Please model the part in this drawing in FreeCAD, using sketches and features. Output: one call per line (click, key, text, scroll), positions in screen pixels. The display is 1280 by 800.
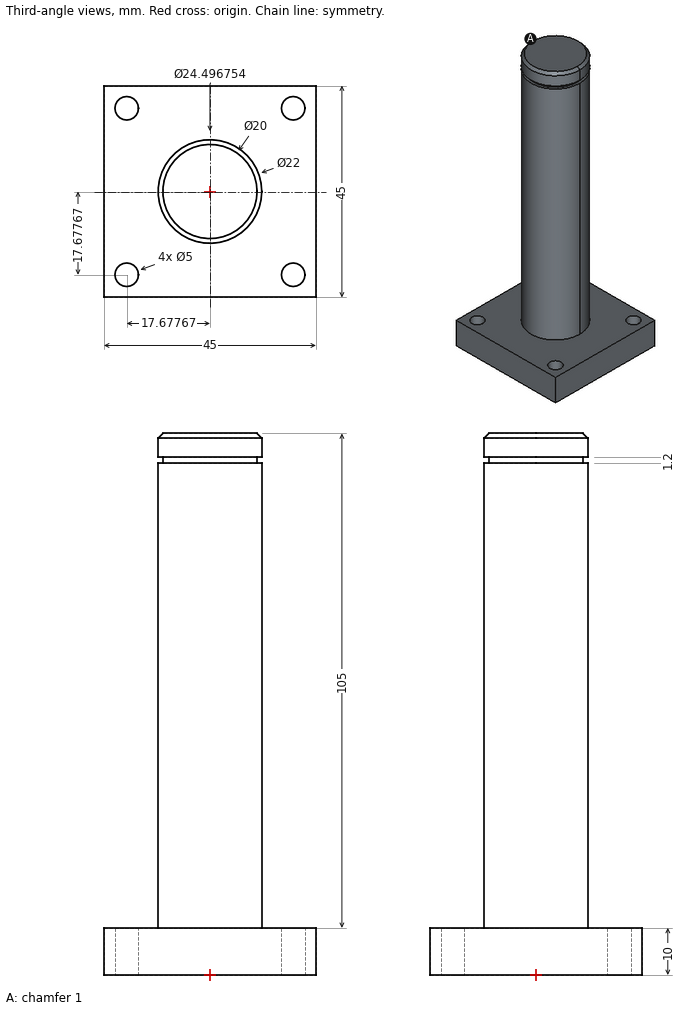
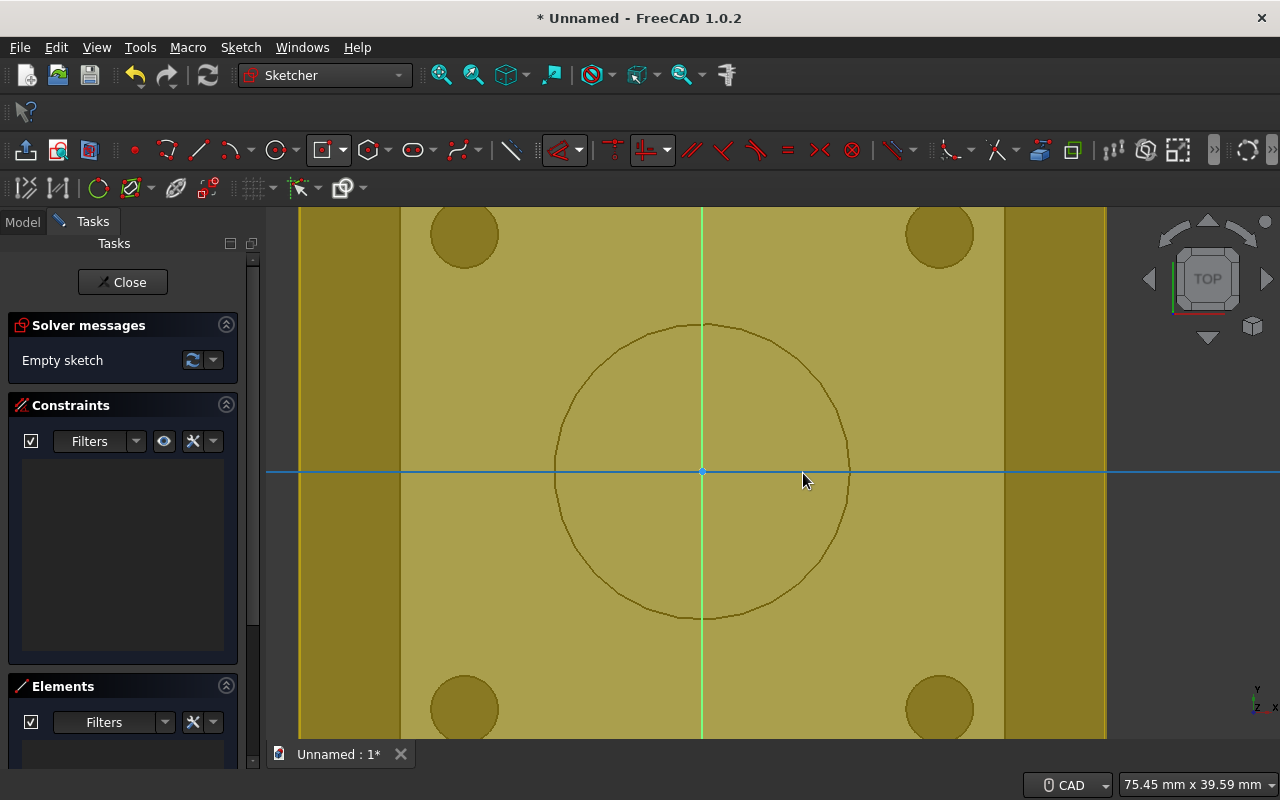
click(276, 150)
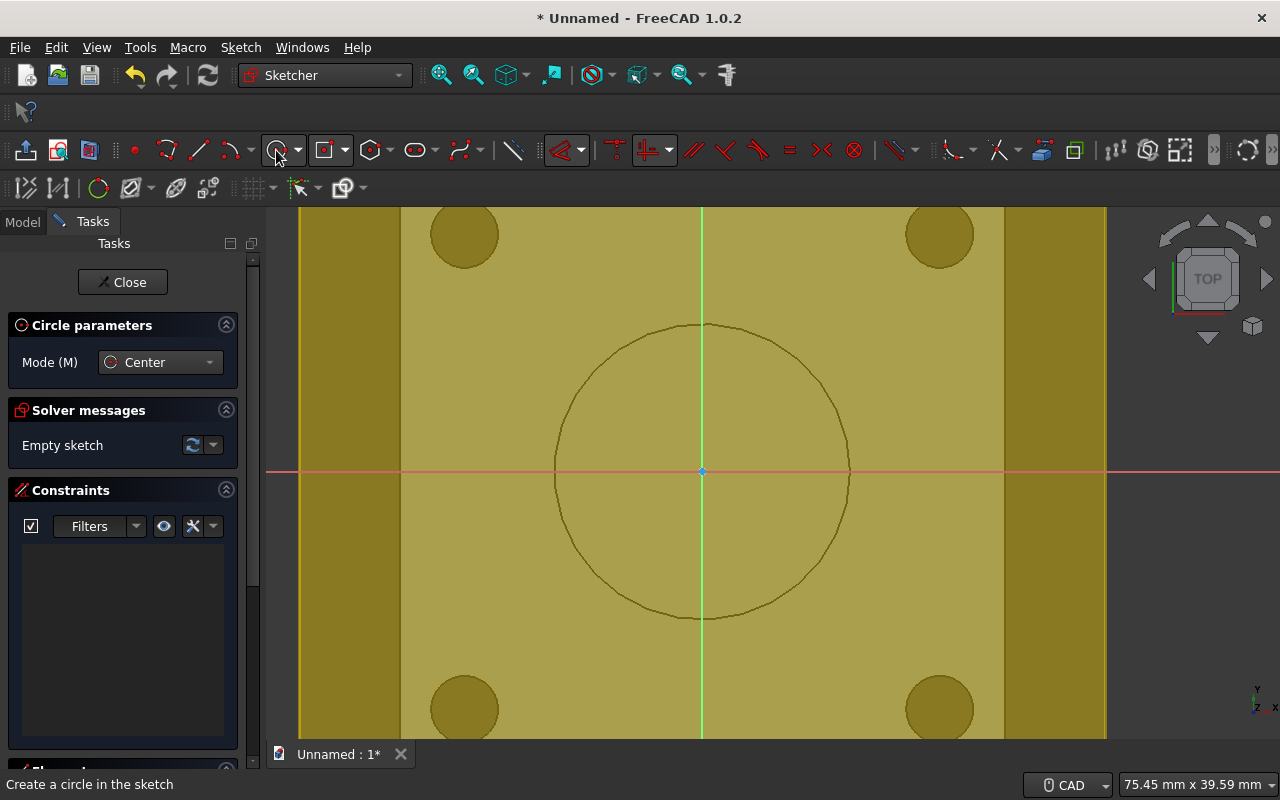
click(702, 472)
move(819, 355)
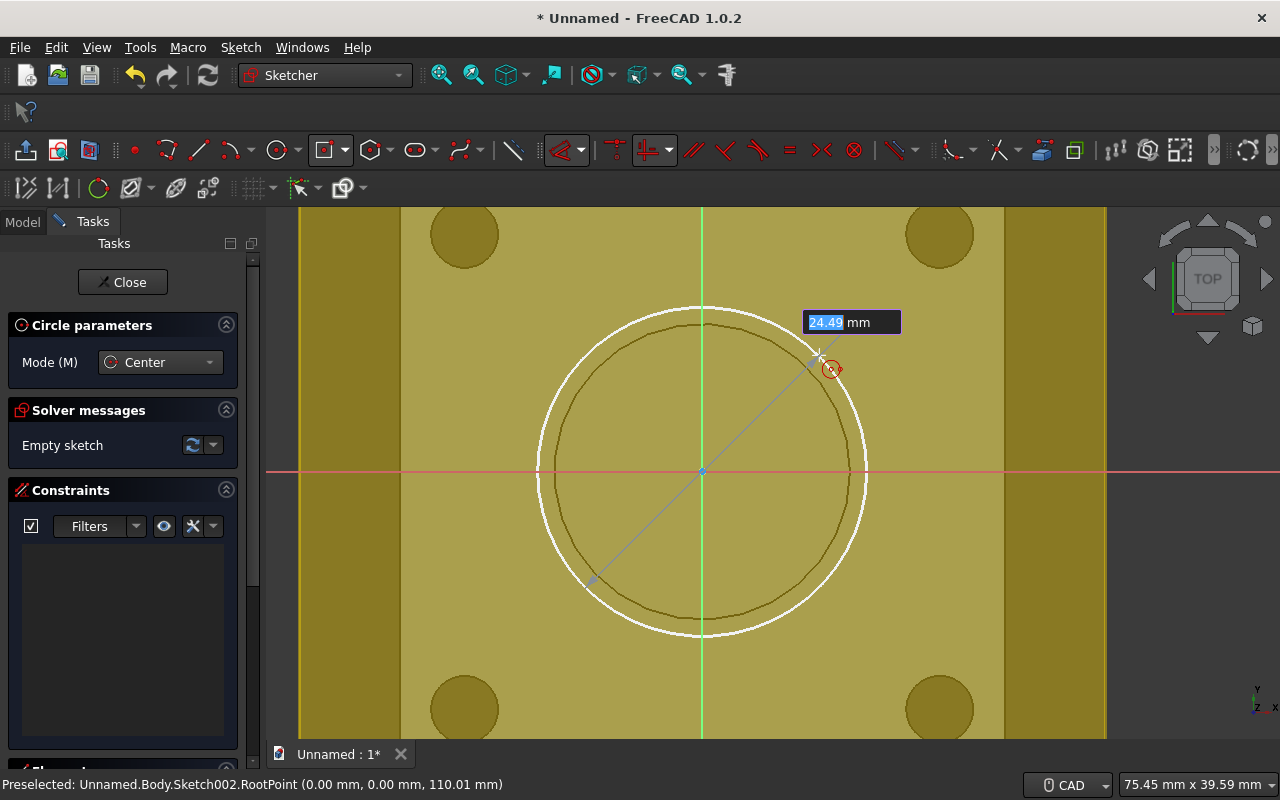
text(24.496754)
key(Return)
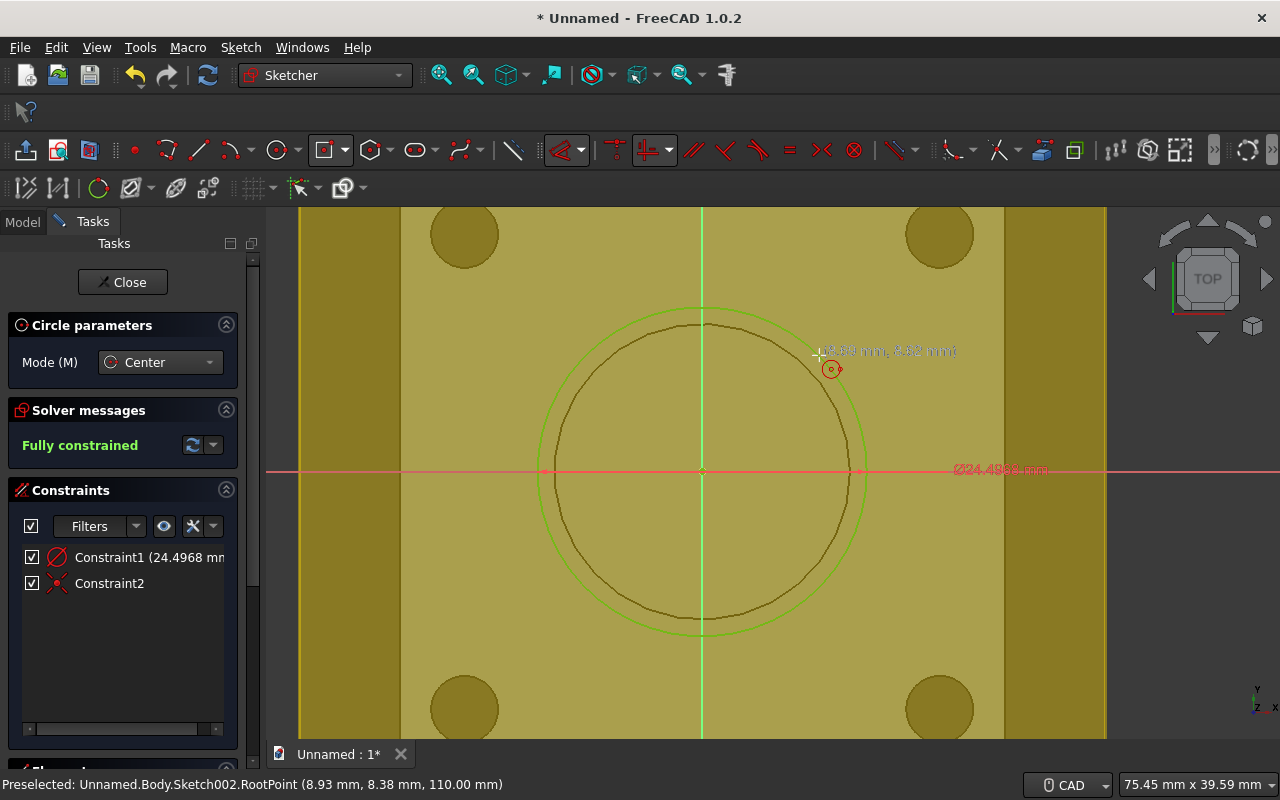
click(702, 472)
move(797, 377)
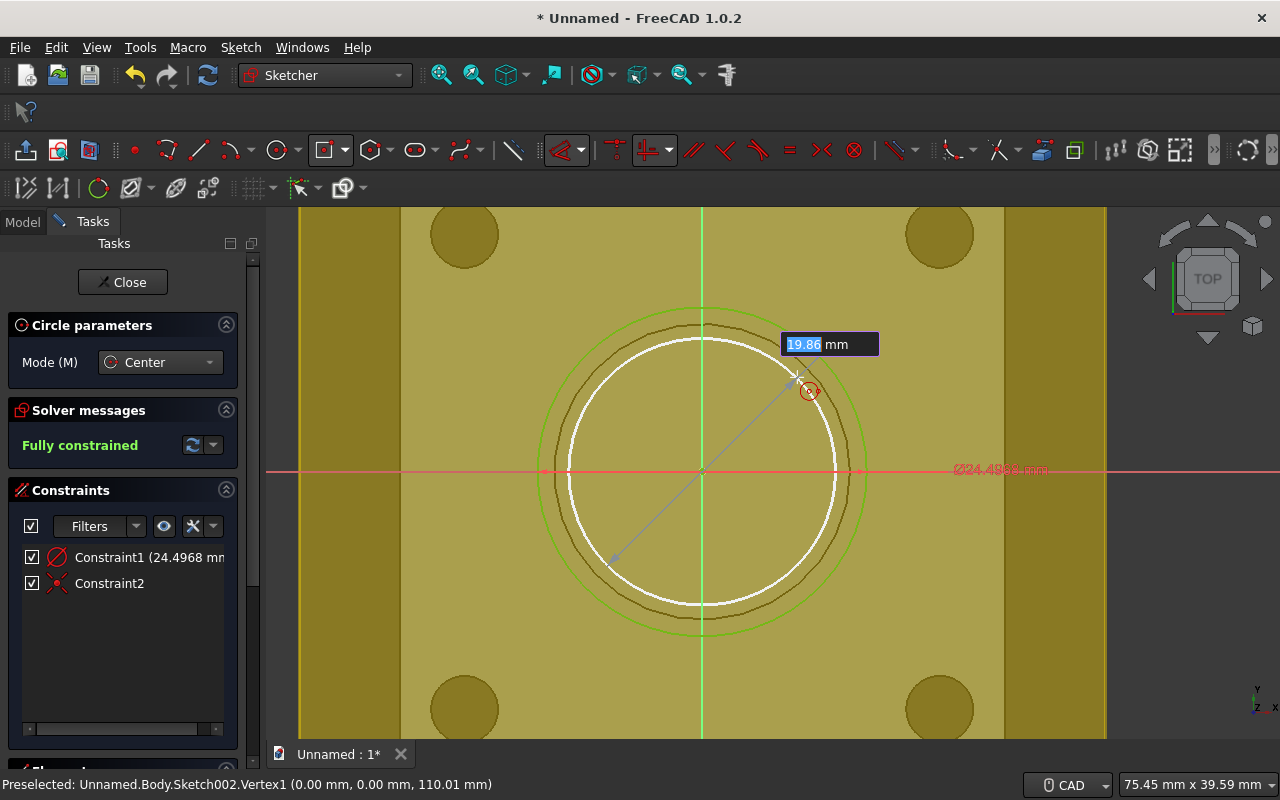
text(20)
key(Return)
key(Escape)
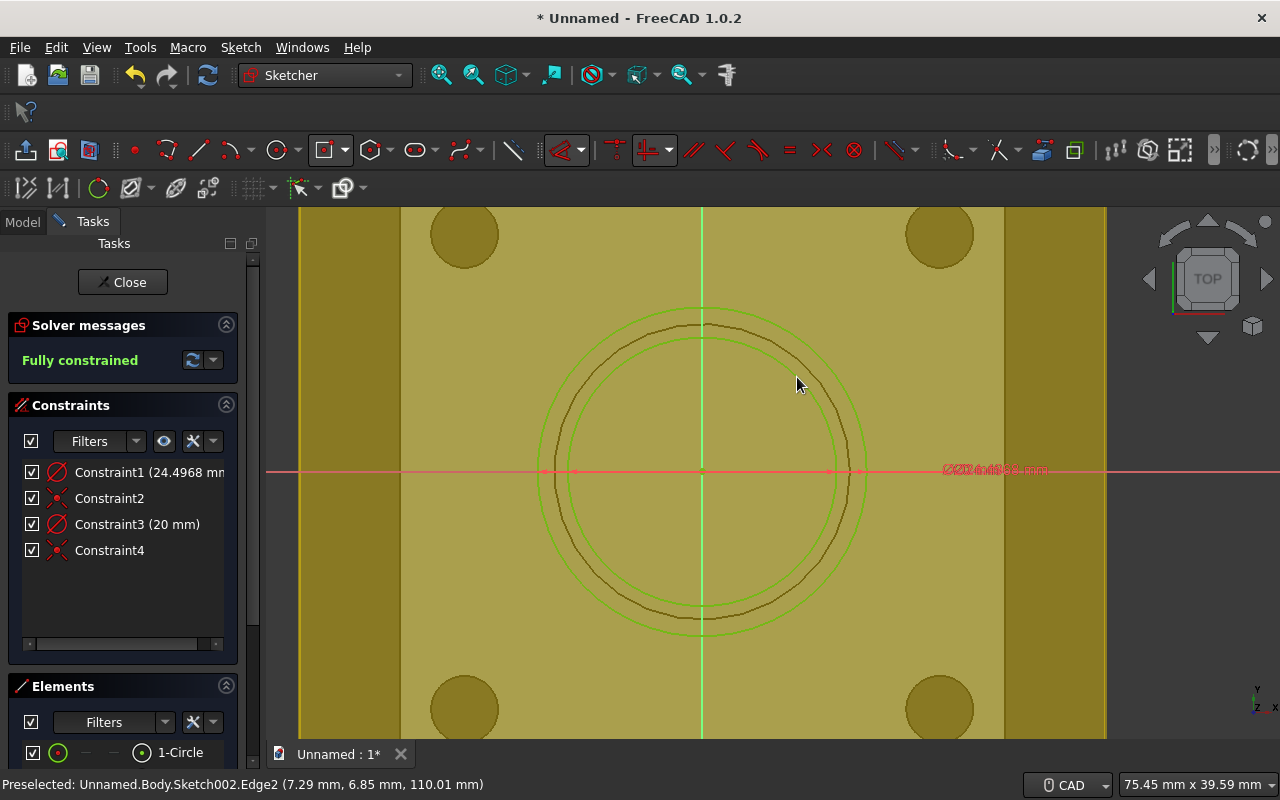
click(123, 282)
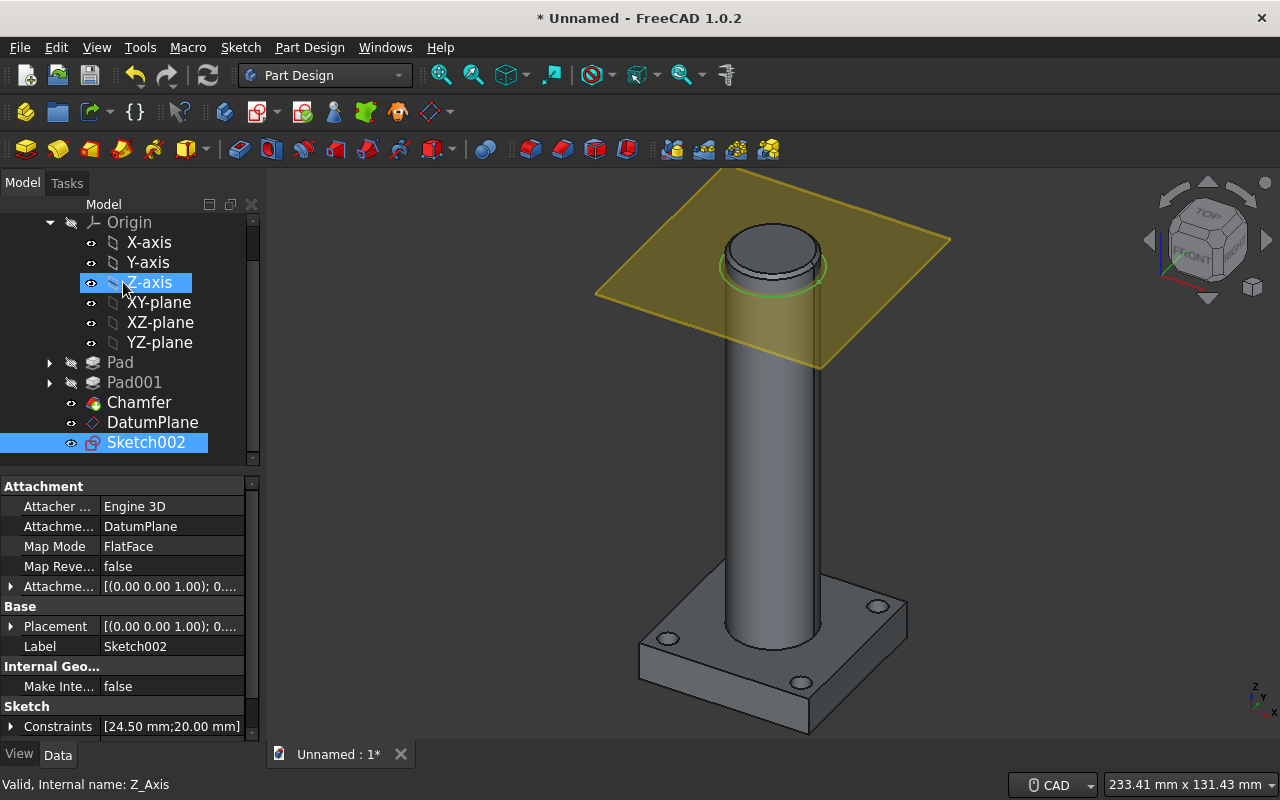
click(240, 150)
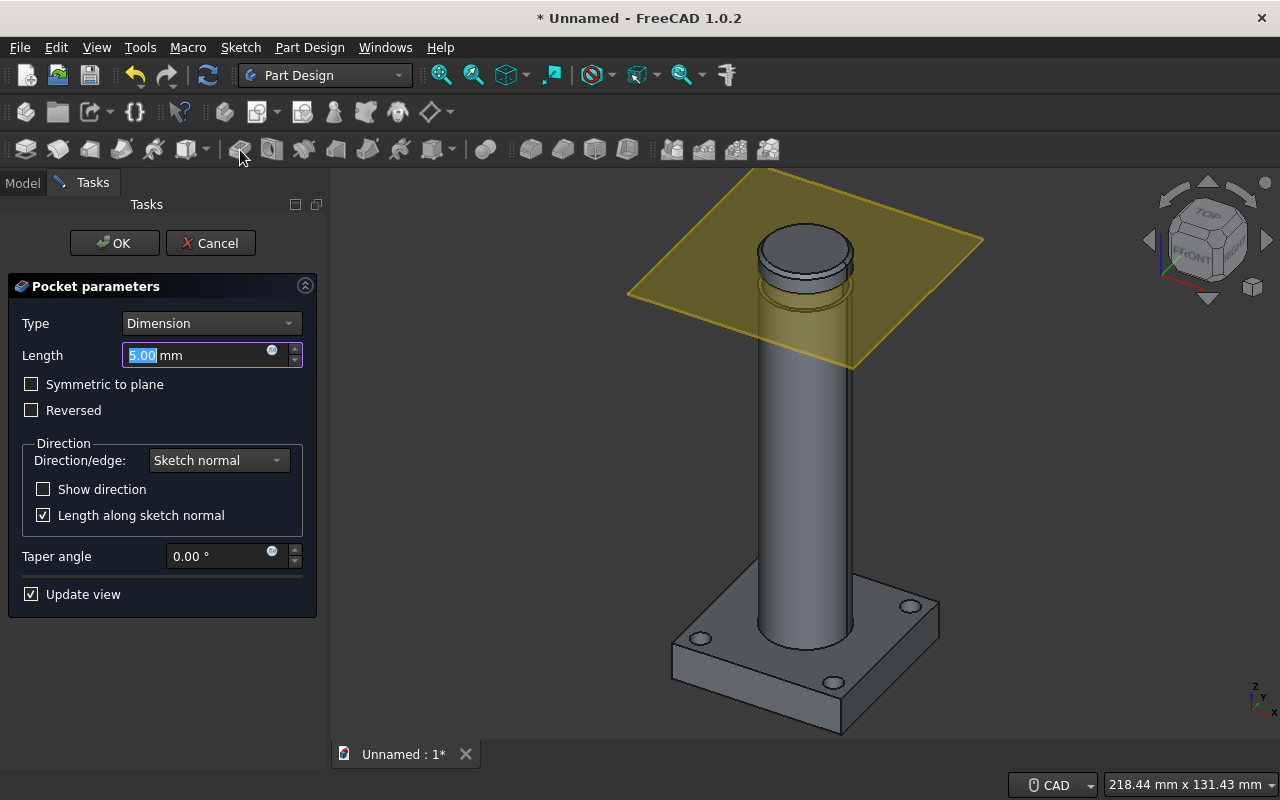
text(1.2)
key(Tab)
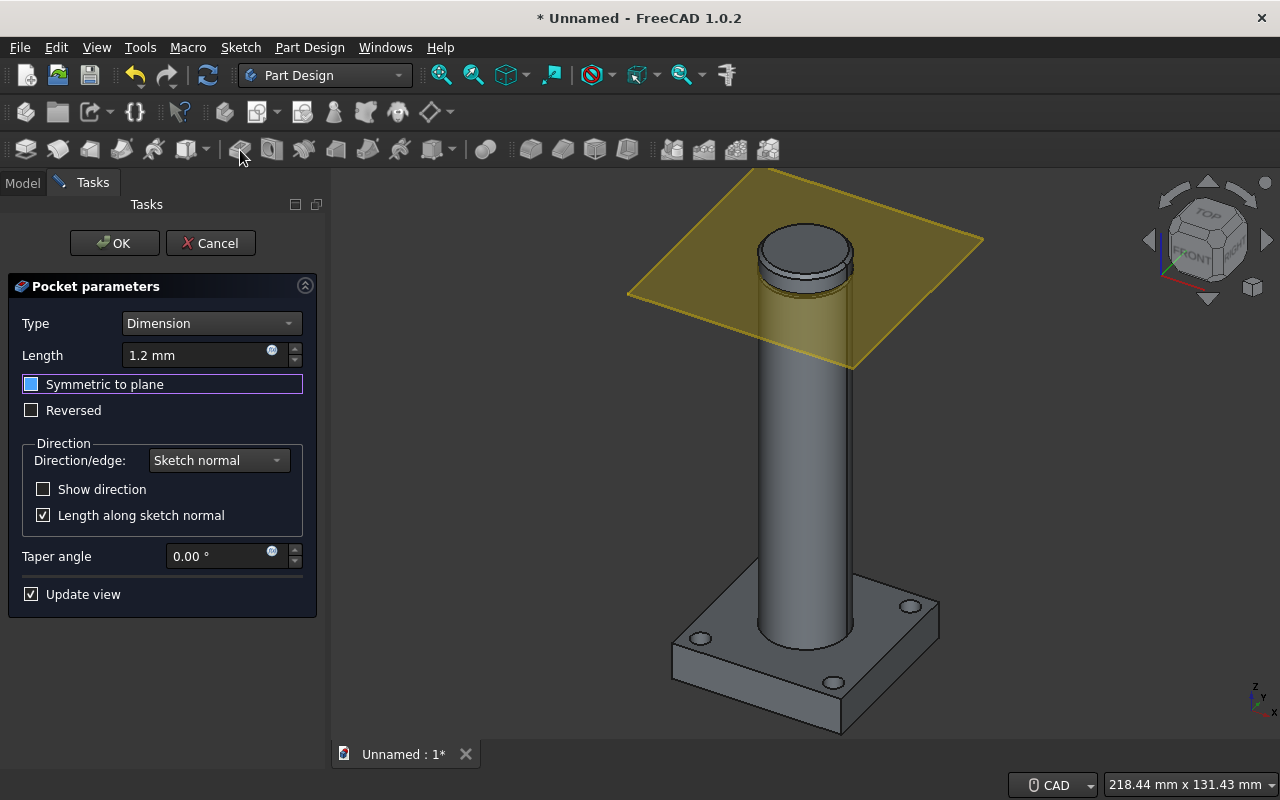
click(115, 243)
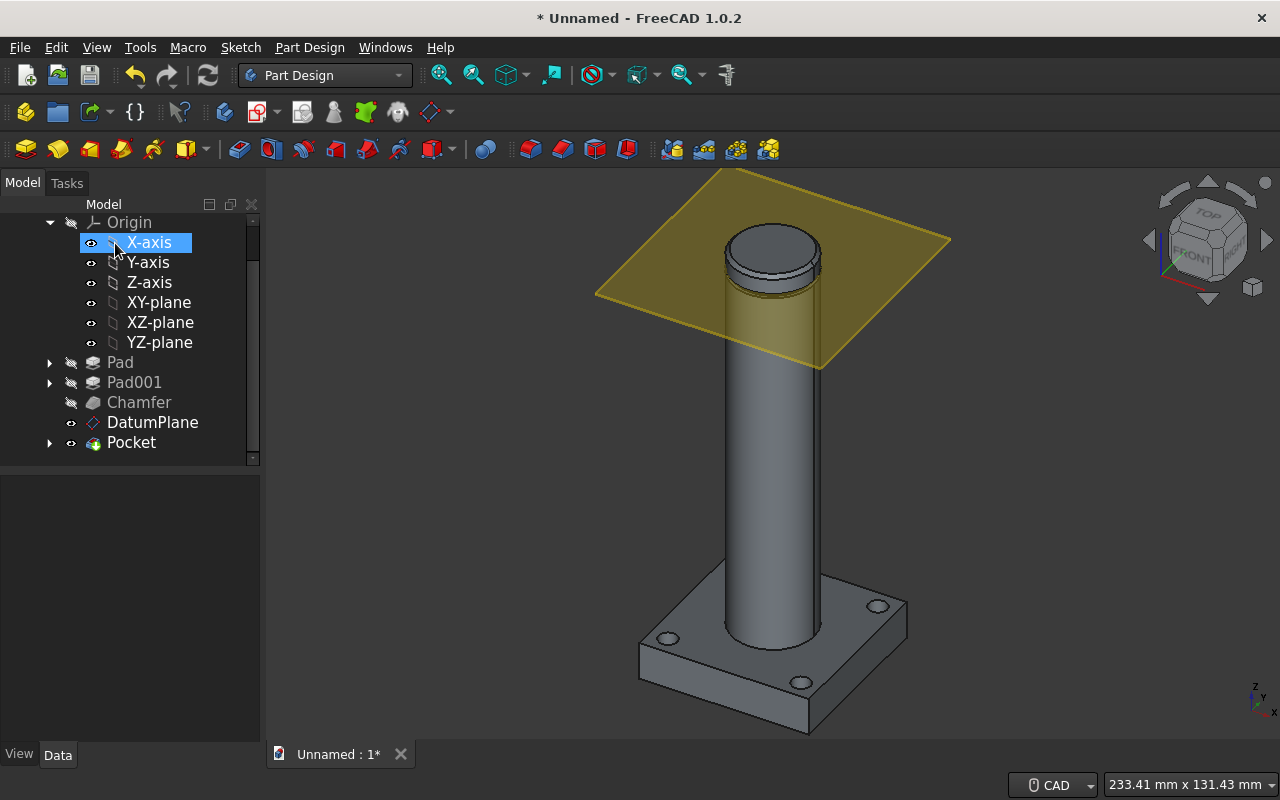
click(116, 423)
key(space)